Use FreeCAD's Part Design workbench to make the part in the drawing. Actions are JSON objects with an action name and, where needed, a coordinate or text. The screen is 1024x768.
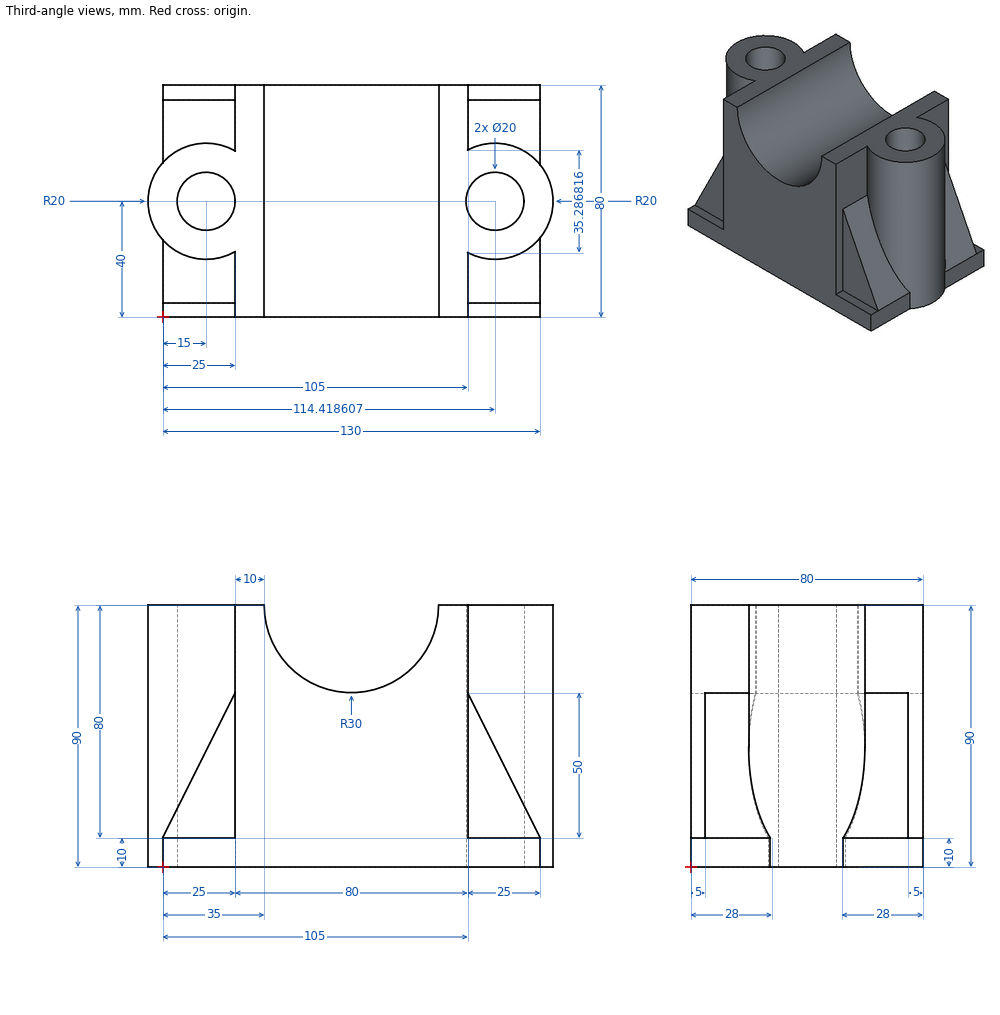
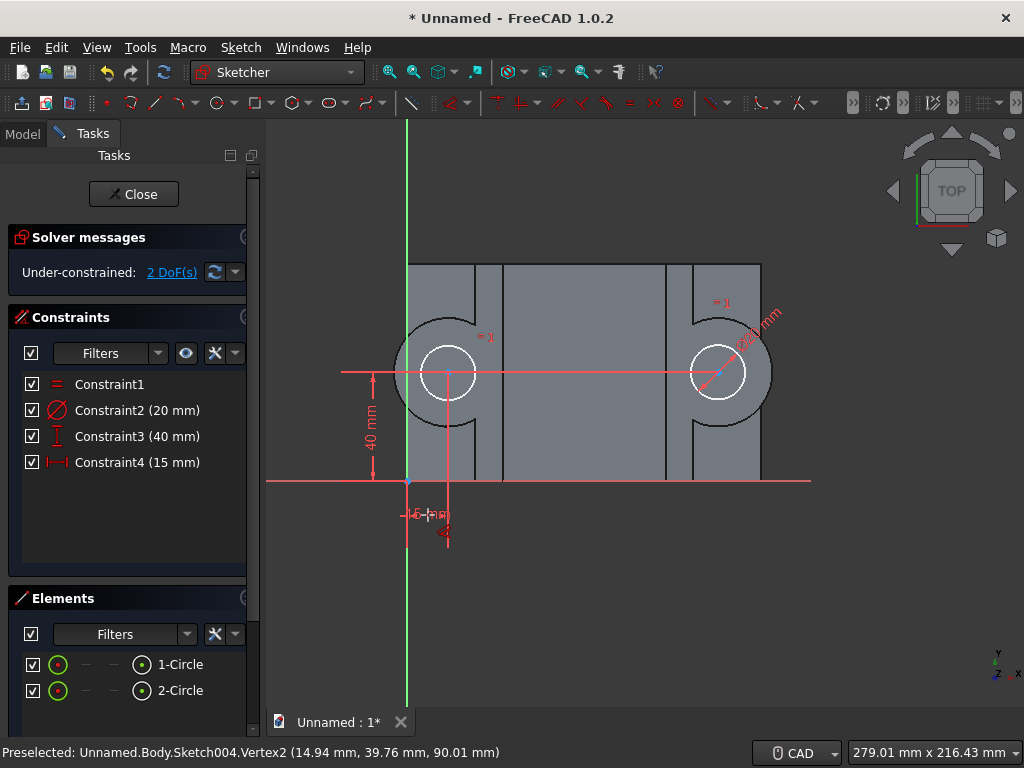
{"action": "left_click", "coordinate": [448, 373]}
{"action": "left_click", "coordinate": [373, 402]}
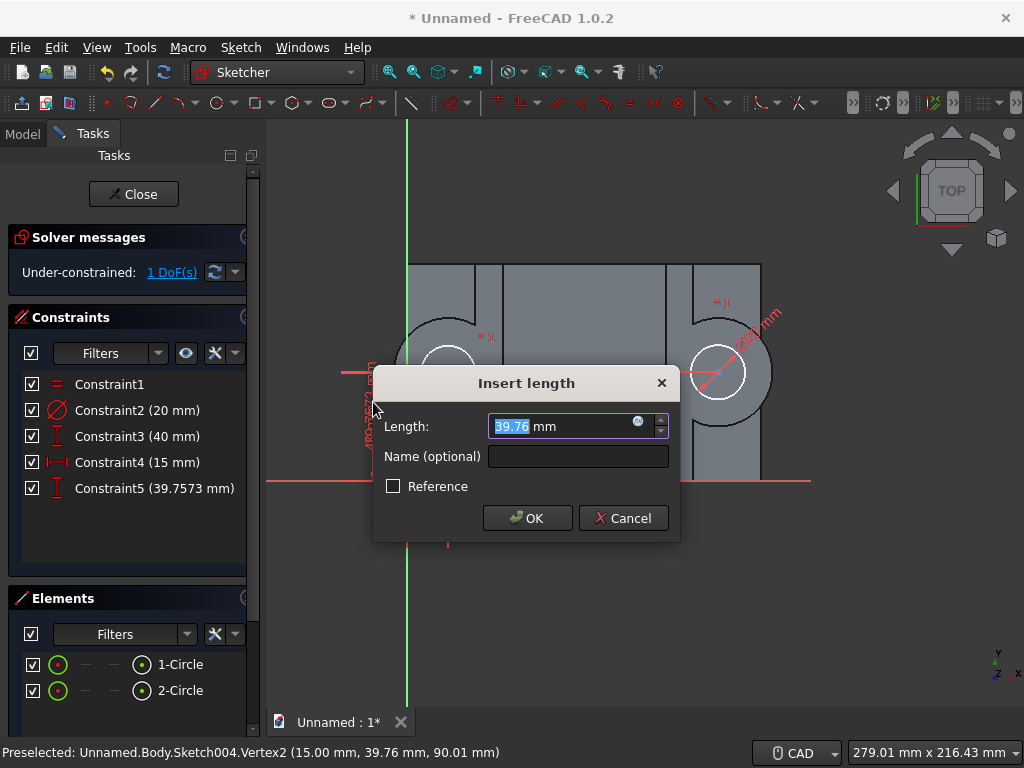
{"action": "type", "text": "40"}
{"action": "key", "text": "Return"}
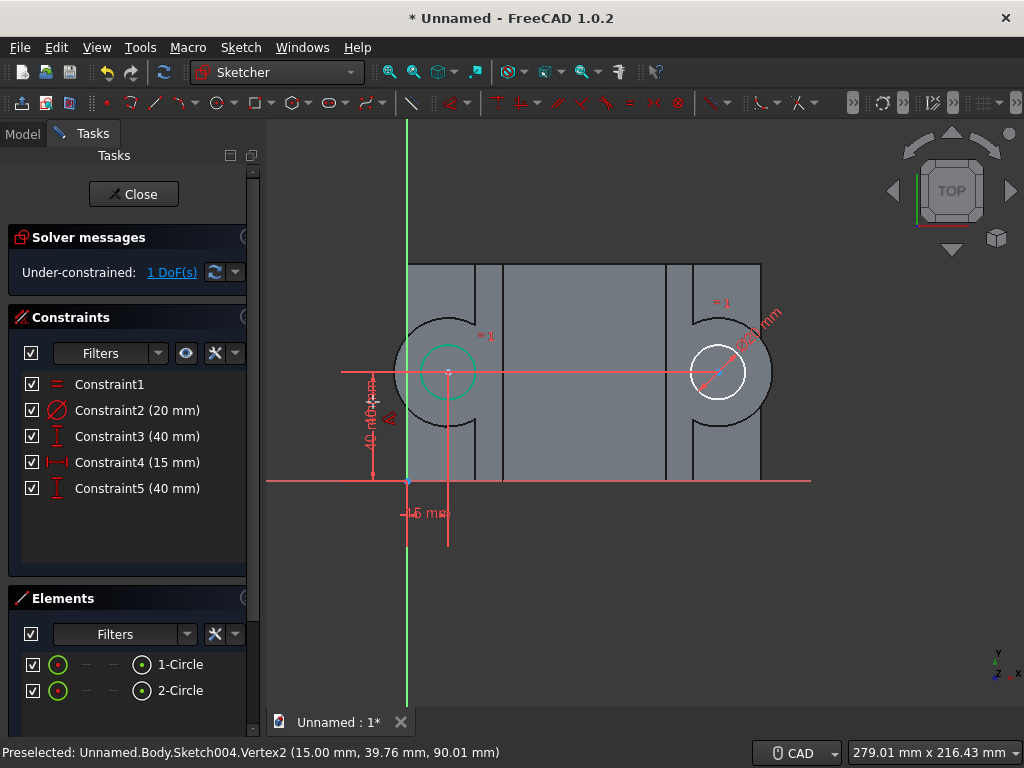
{"action": "left_click", "coordinate": [718, 372]}
{"action": "left_click", "coordinate": [563, 515]}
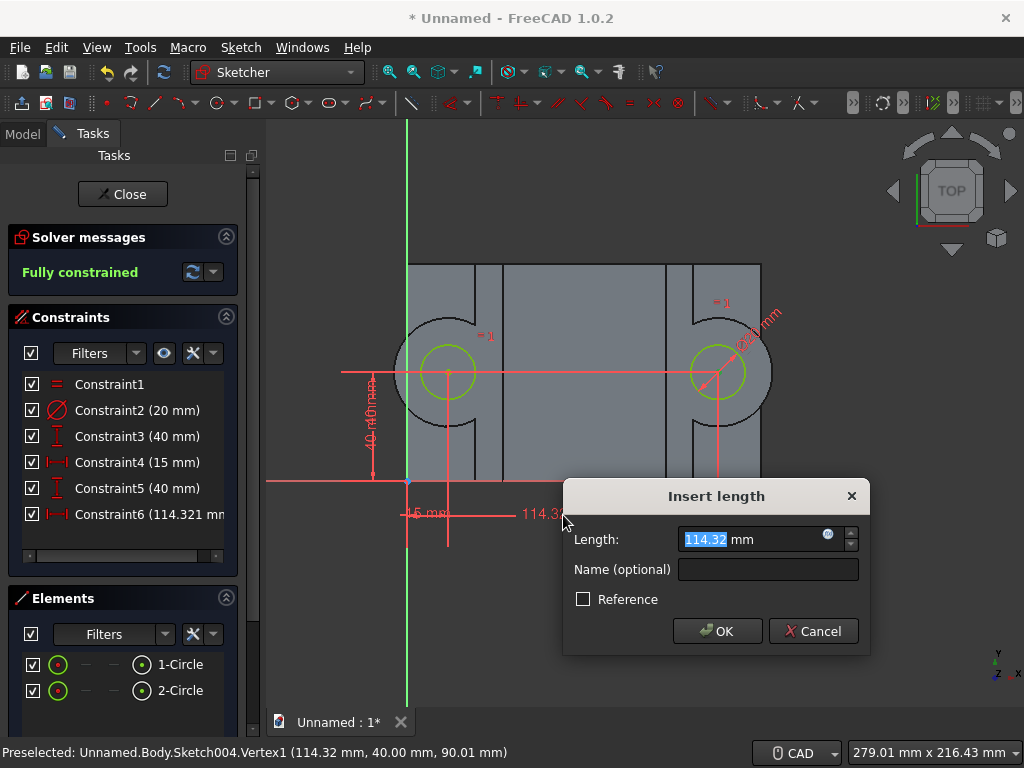
{"action": "type", "text": "114.418607"}
{"action": "key", "text": "Return"}
{"action": "key", "text": "Escape"}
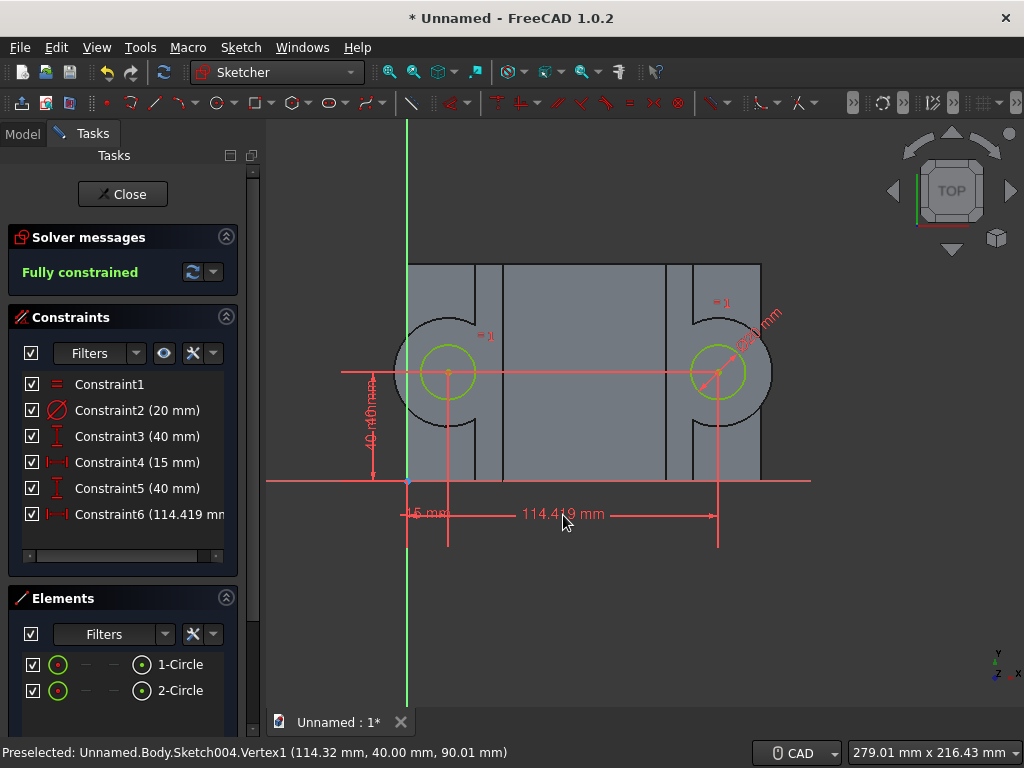
{"action": "left_click", "coordinate": [123, 194]}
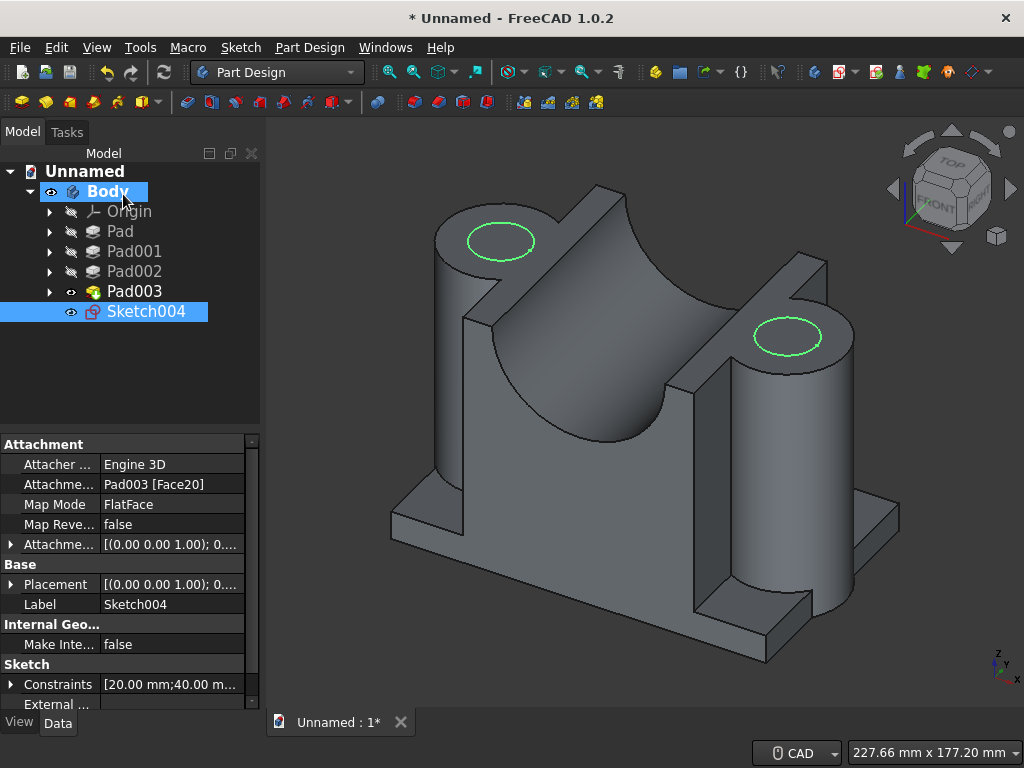
{"action": "left_click", "coordinate": [188, 102]}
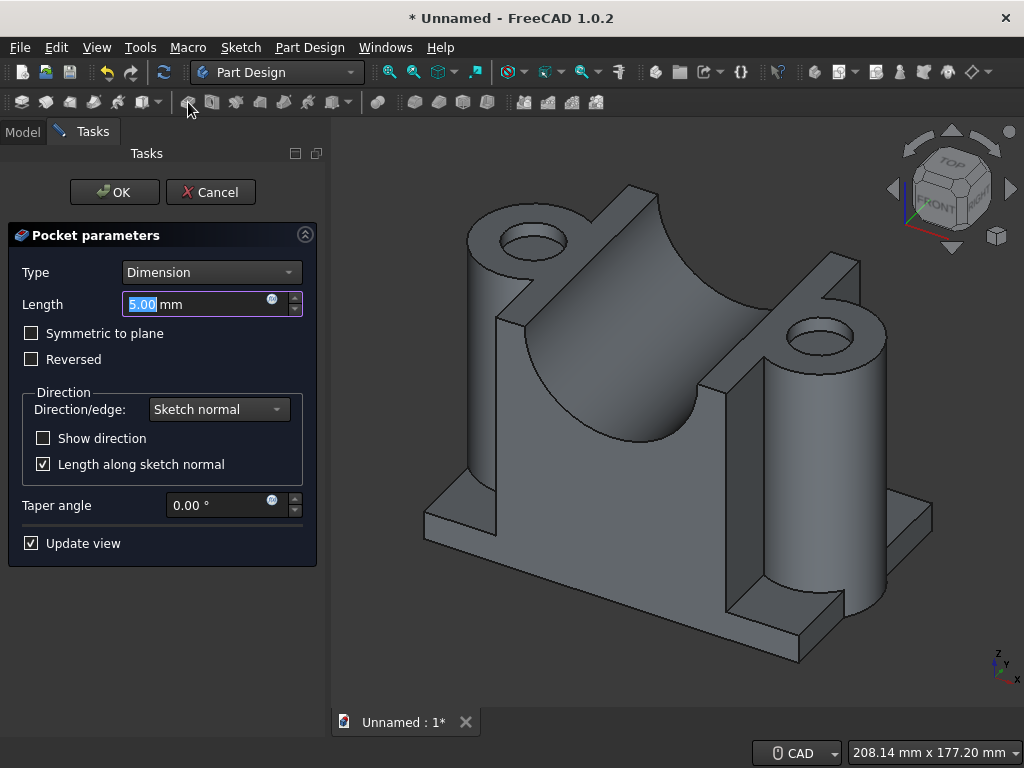
{"action": "type", "text": "90"}
{"action": "key", "text": "Tab"}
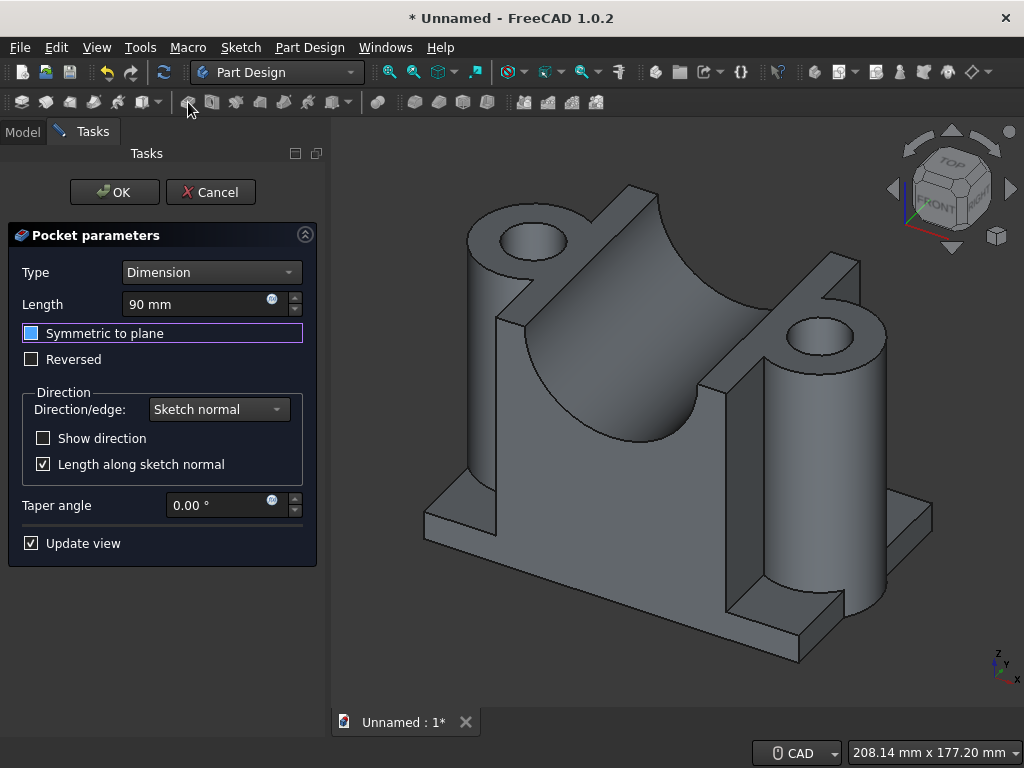
{"action": "left_click", "coordinate": [115, 192]}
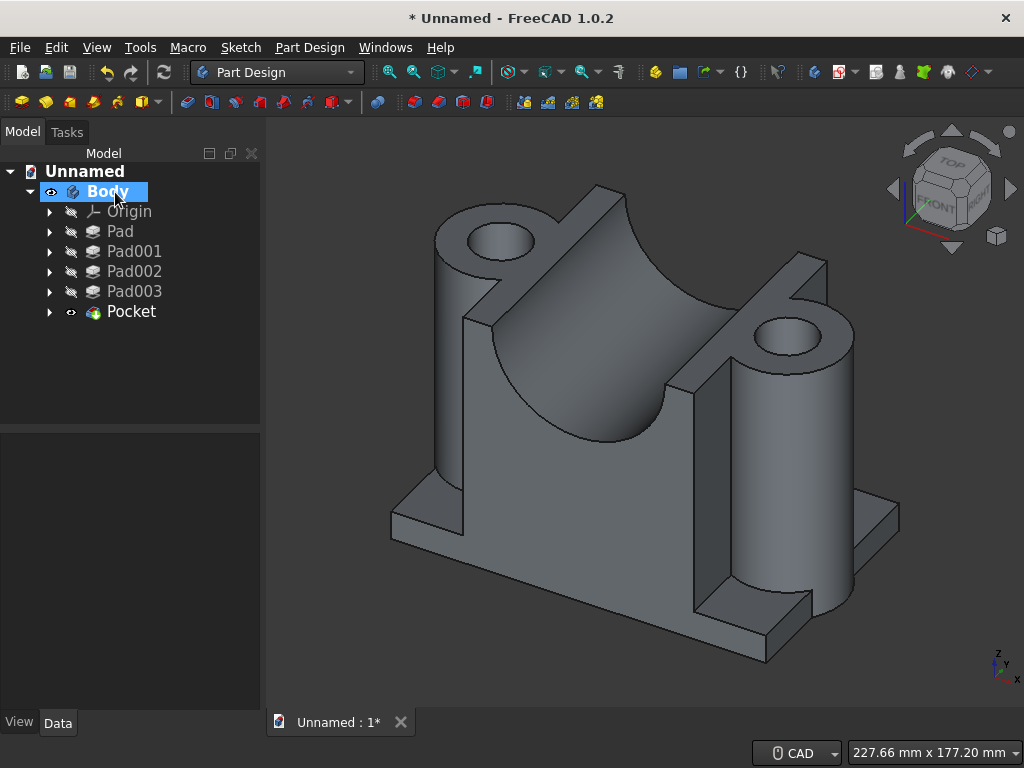
{"action": "left_click", "coordinate": [579, 512]}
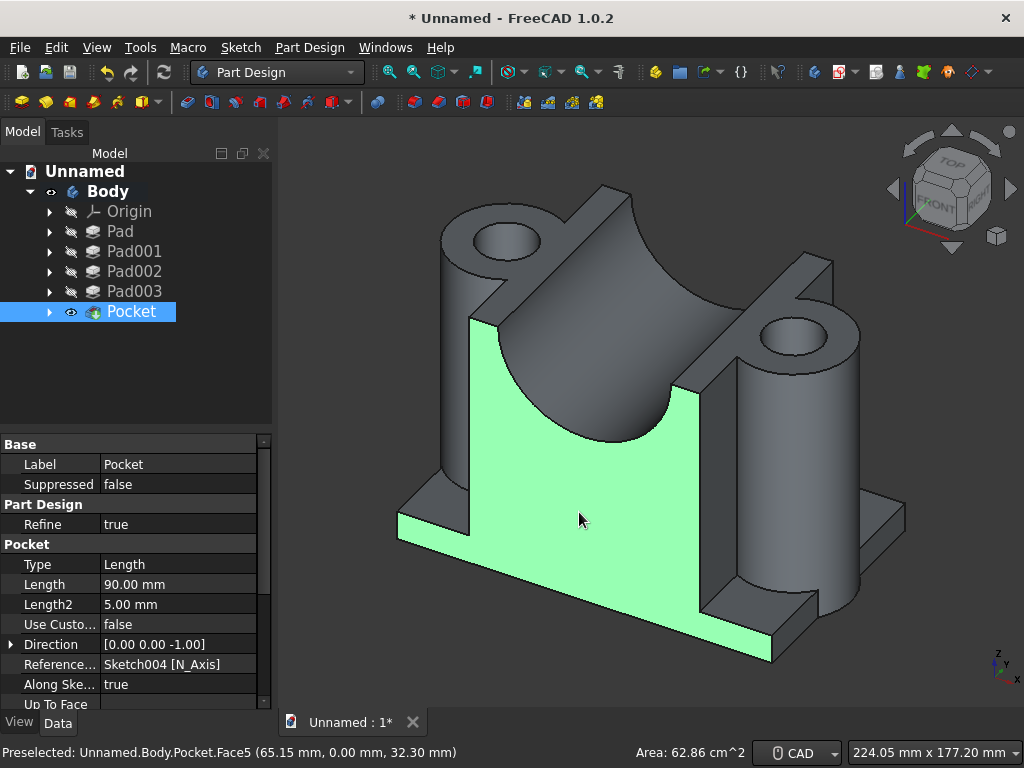
{"action": "left_click", "coordinate": [840, 72]}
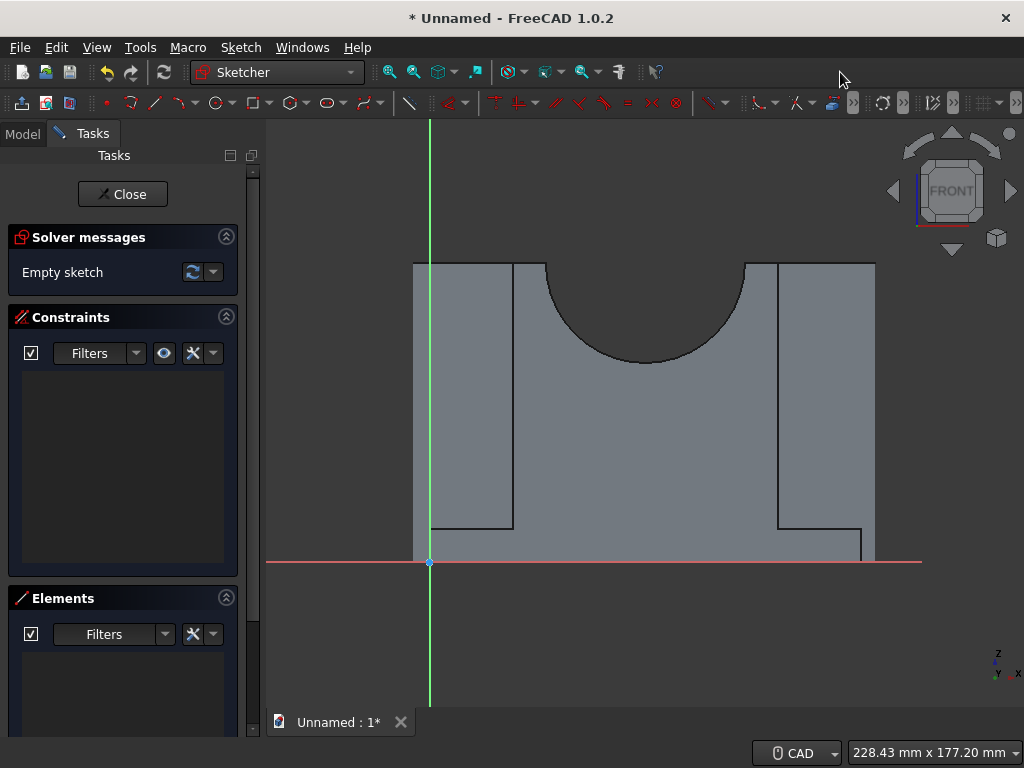
{"action": "scroll", "coordinate": [576, 413], "scroll_direction": "down", "scroll_amount": 5}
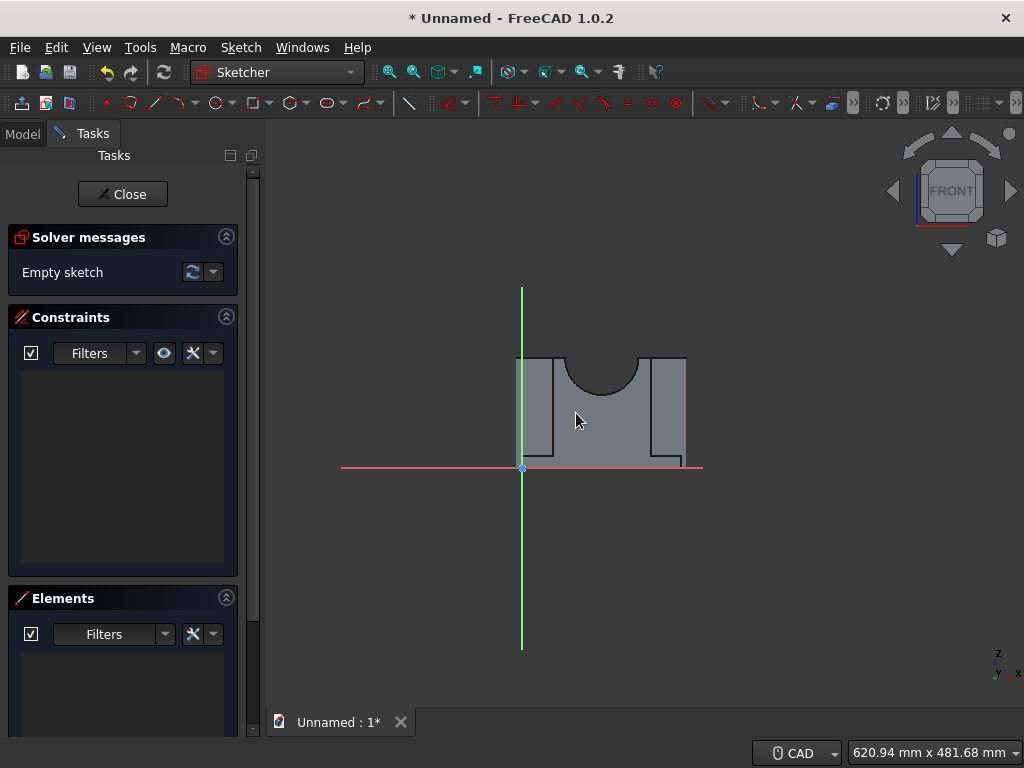
{"action": "scroll", "coordinate": [684, 428], "scroll_direction": "up", "scroll_amount": 9}